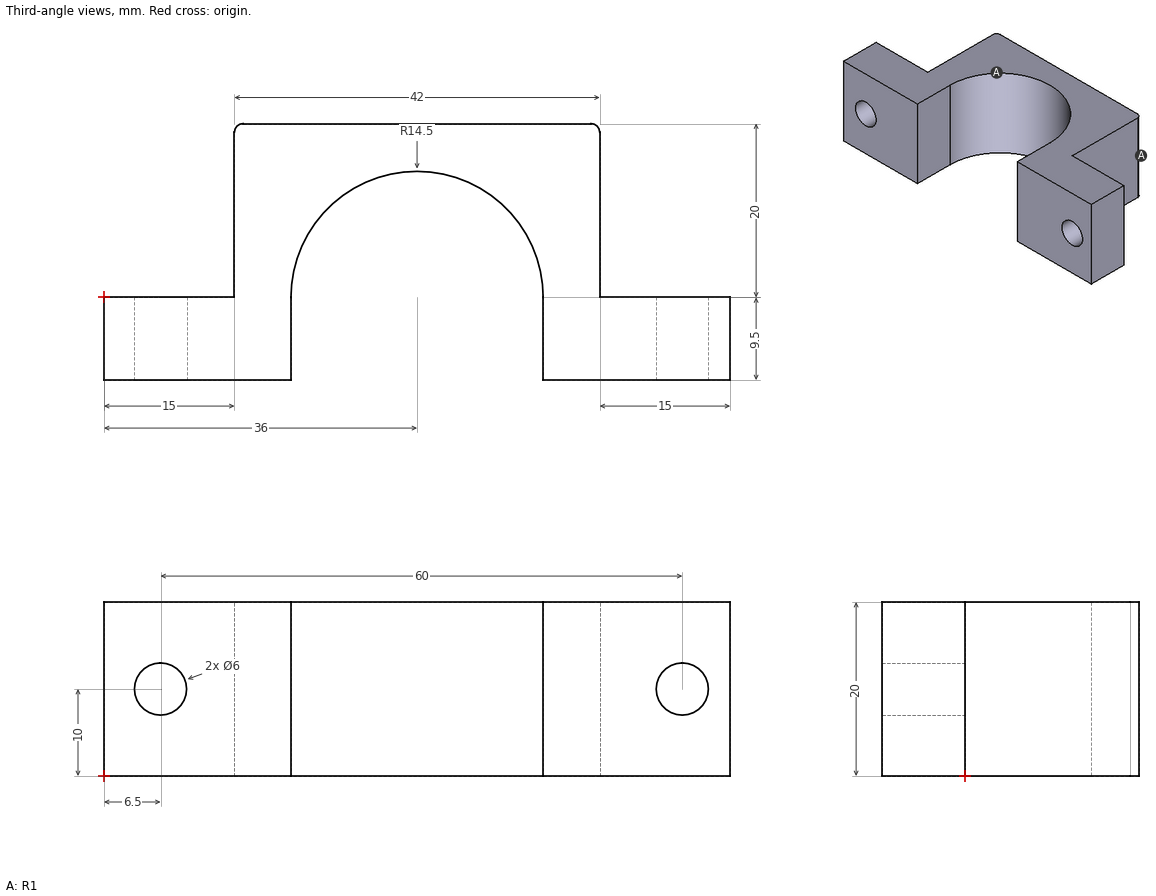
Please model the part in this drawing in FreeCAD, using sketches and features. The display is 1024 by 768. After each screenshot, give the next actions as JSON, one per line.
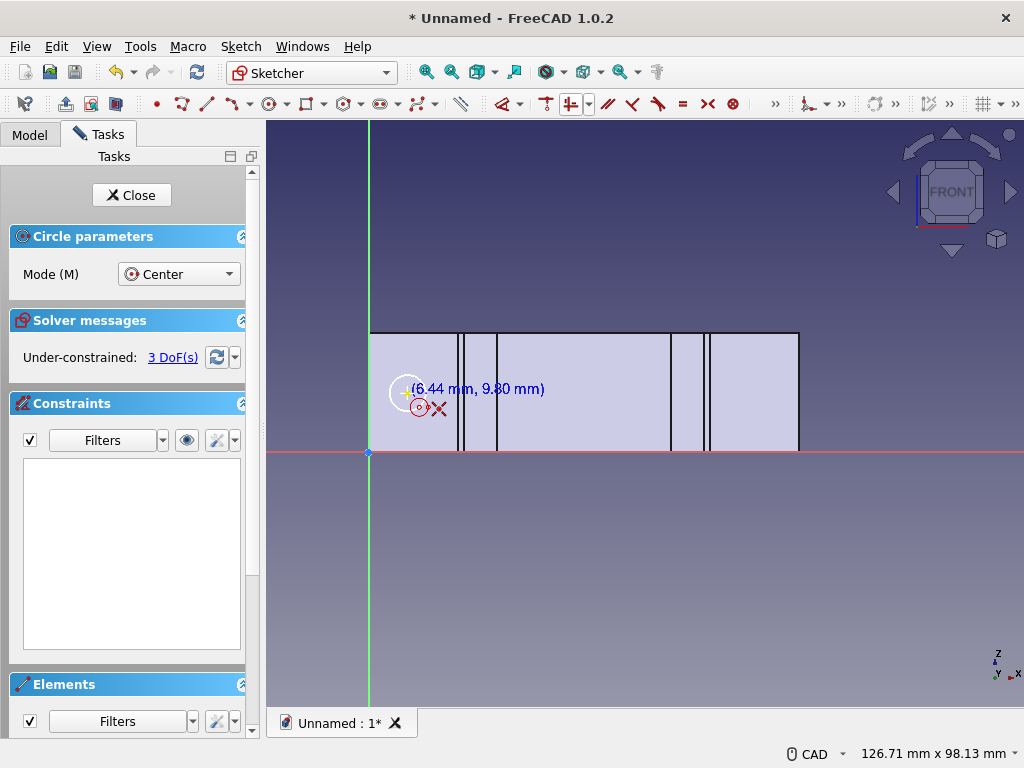
{"action": "scroll", "coordinate": [766, 393], "scroll_direction": "up", "scroll_amount": 2}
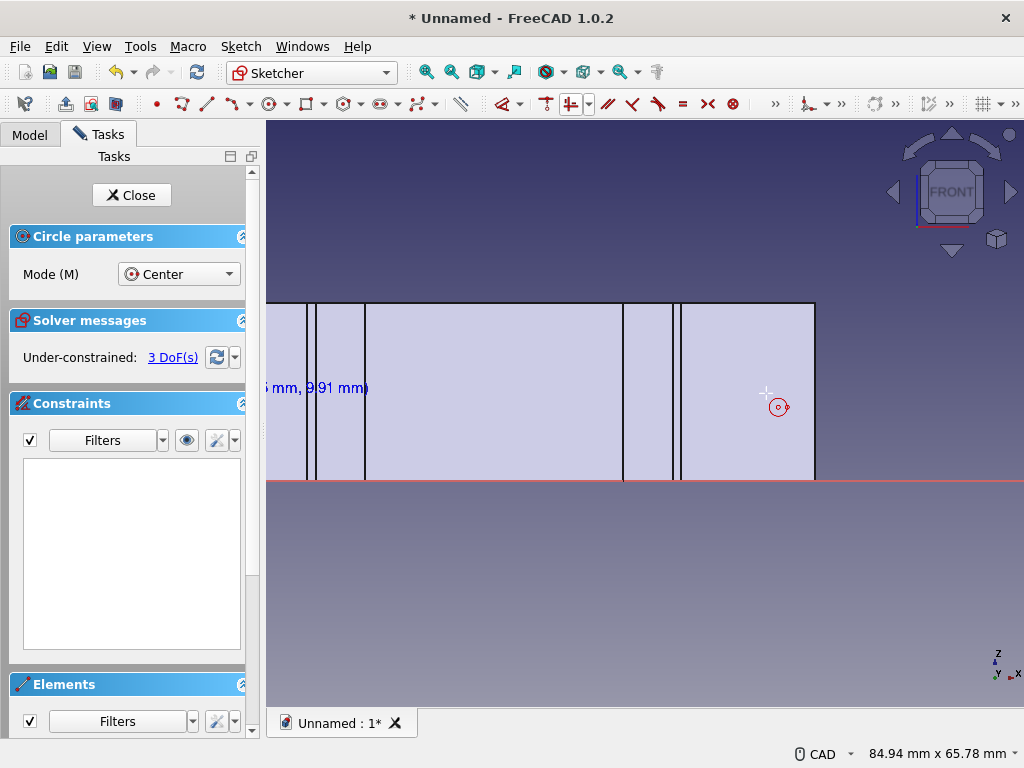
{"action": "left_click", "coordinate": [766, 392]}
{"action": "left_click", "coordinate": [785, 373]}
{"action": "key", "text": "Escape"}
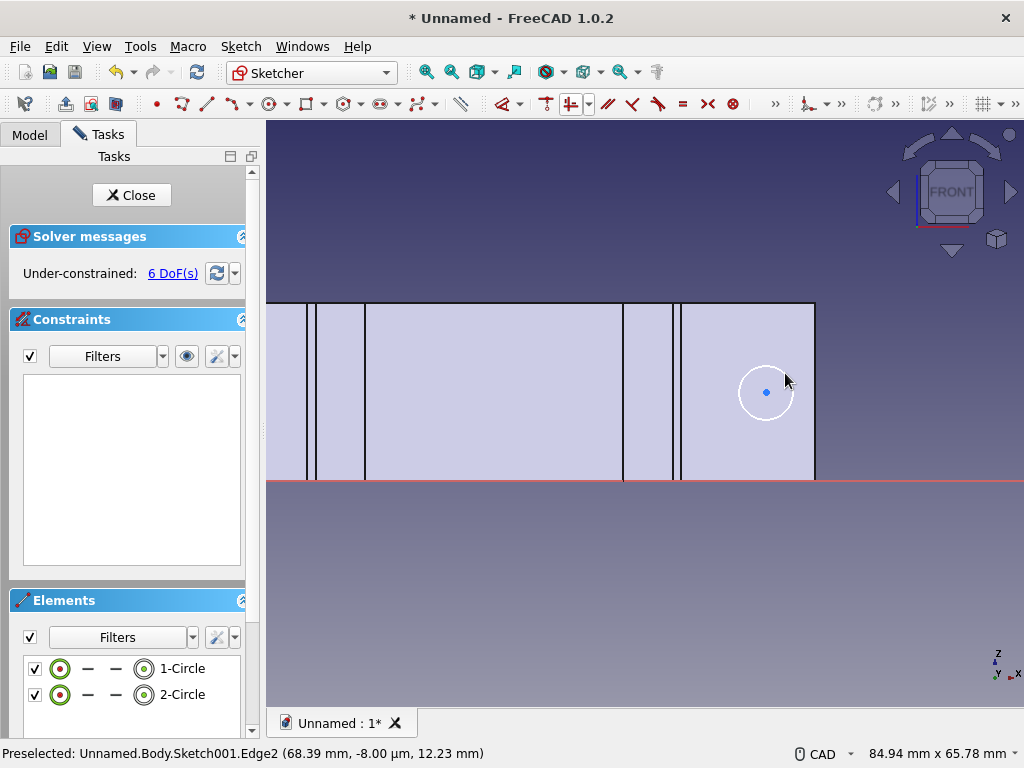
{"action": "scroll", "coordinate": [767, 393], "scroll_direction": "down", "scroll_amount": 2}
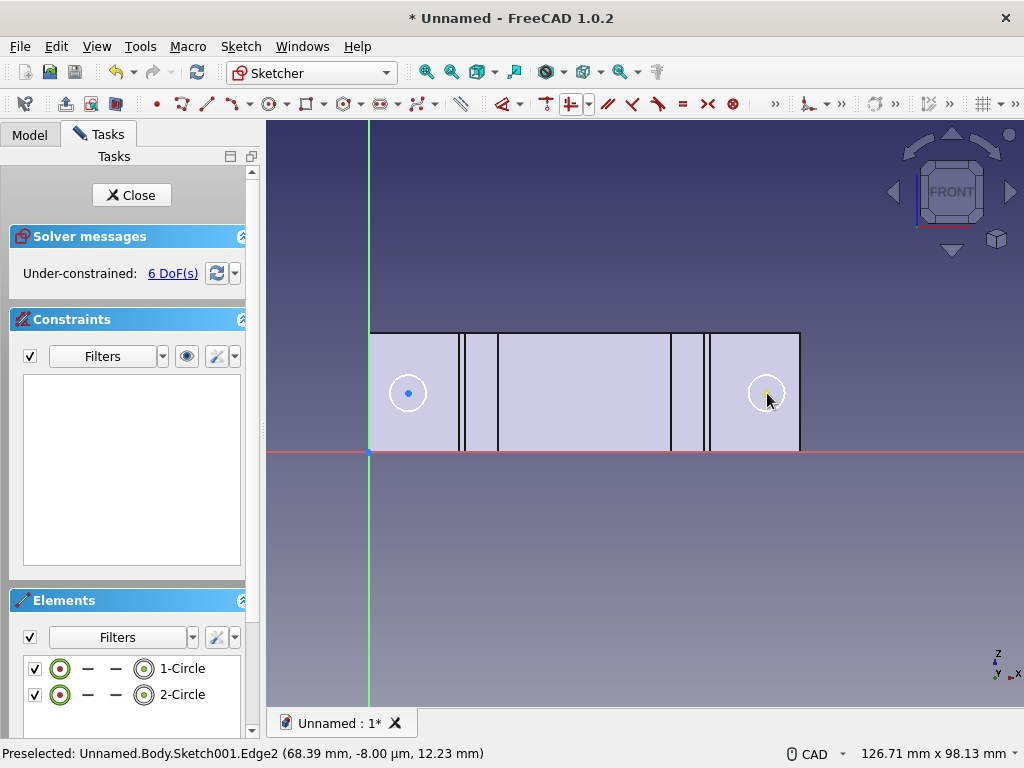
{"action": "left_click", "coordinate": [421, 380]}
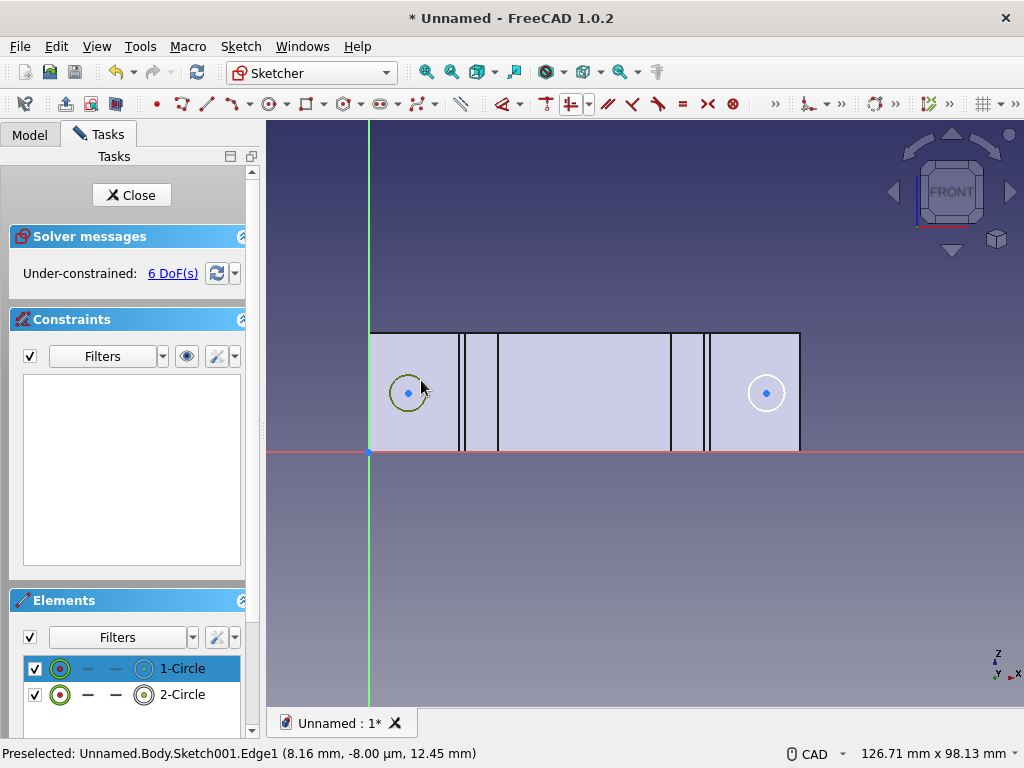
{"action": "left_click", "coordinate": [779, 380]}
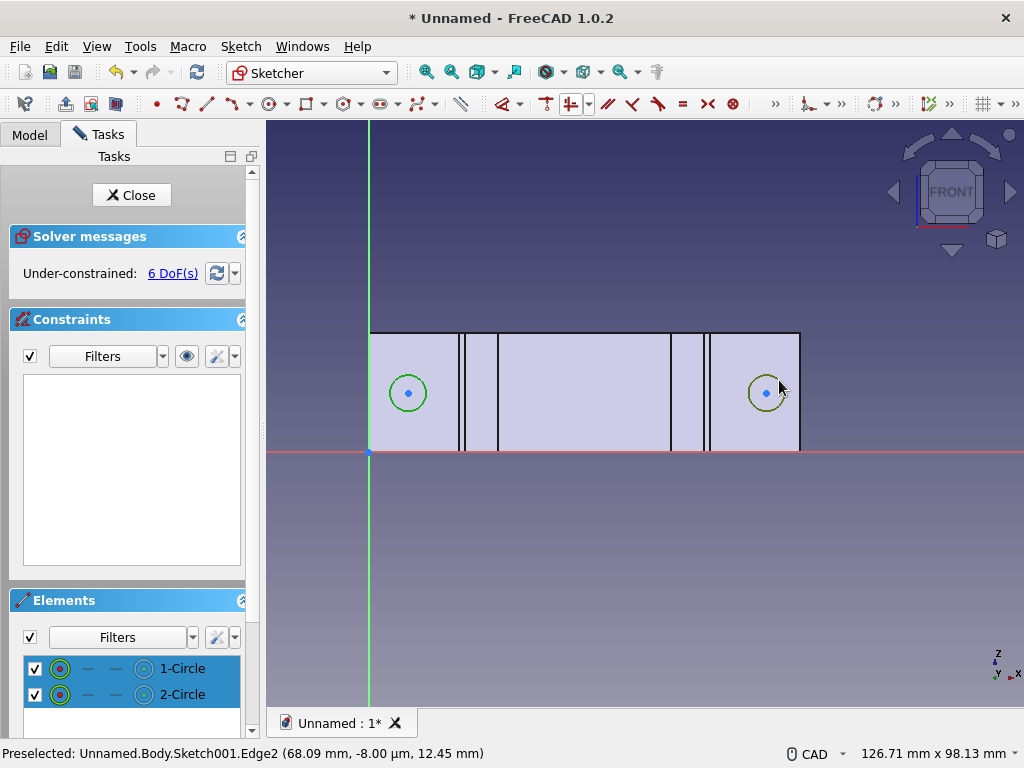
{"action": "left_click", "coordinate": [683, 104]}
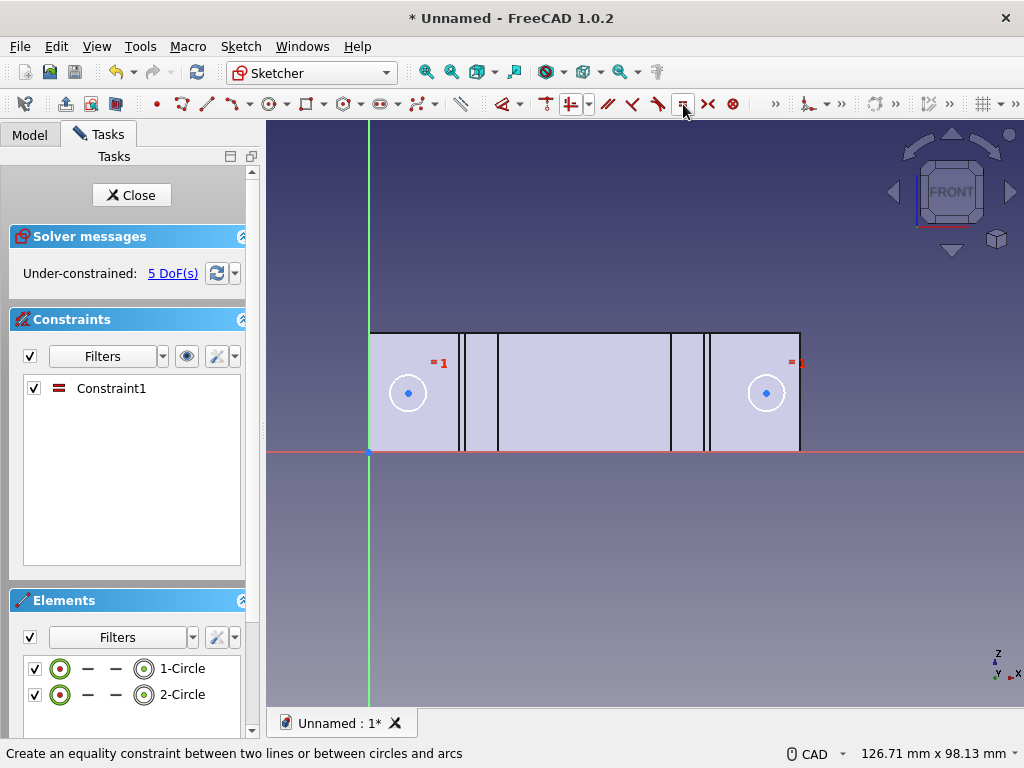
{"action": "left_click", "coordinate": [502, 104]}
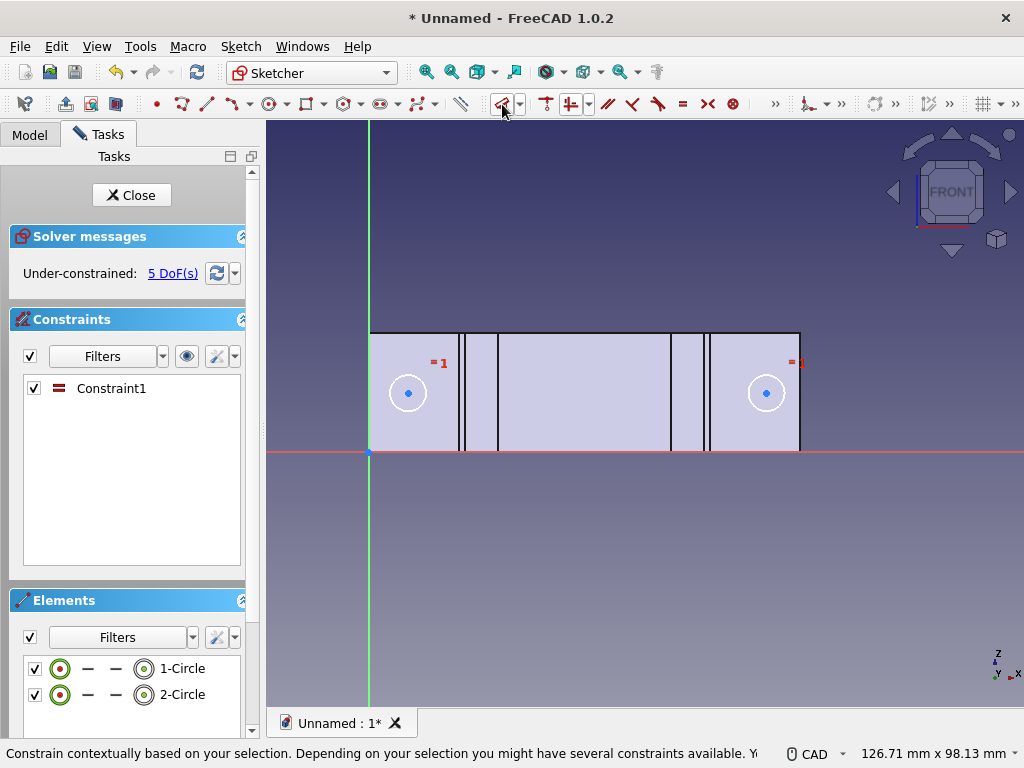
{"action": "left_click", "coordinate": [421, 380]}
{"action": "left_click", "coordinate": [443, 357]}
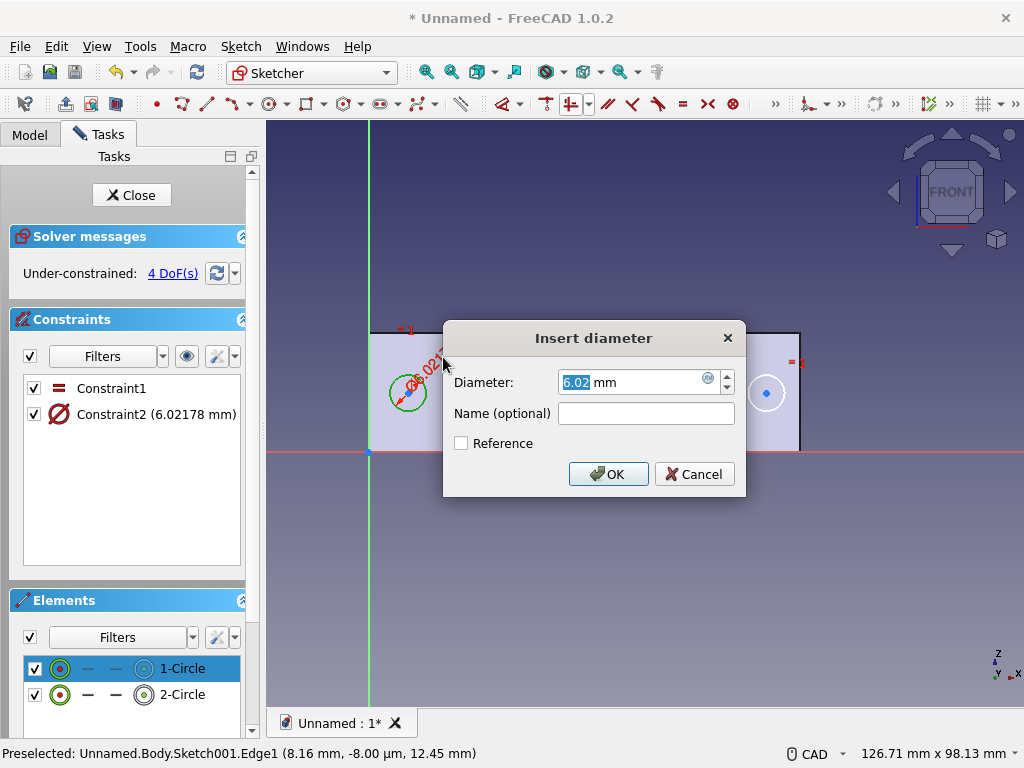
{"action": "type", "text": "6"}
{"action": "key", "text": "Return"}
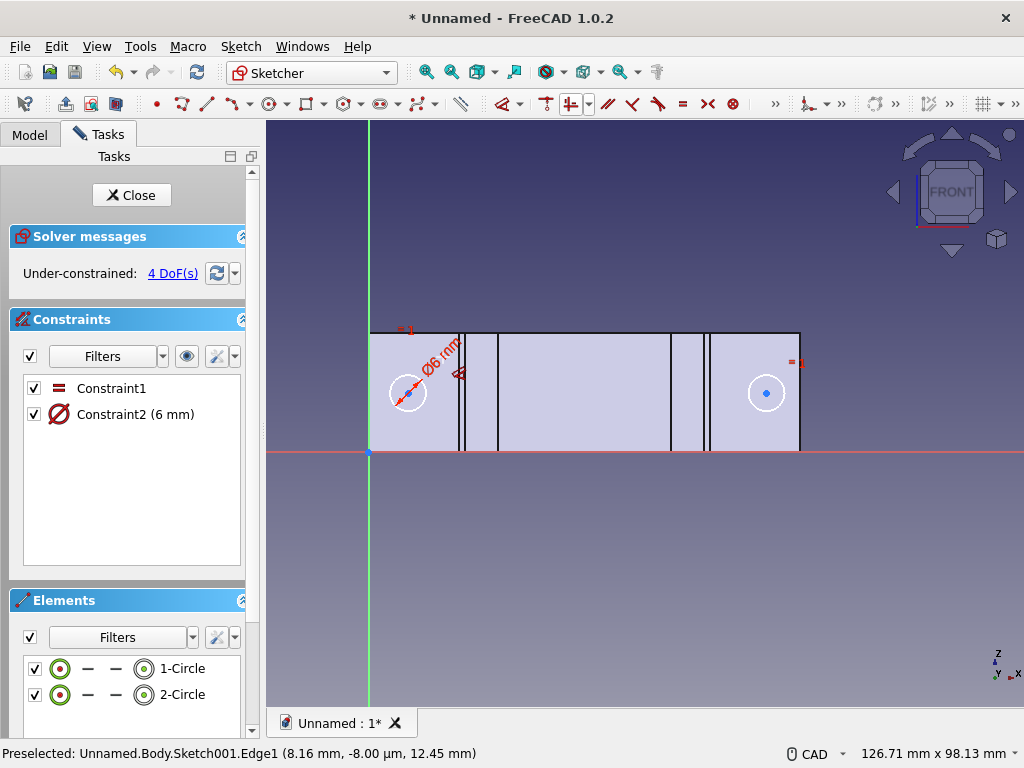
{"action": "left_click", "coordinate": [408, 393]}
{"action": "left_click", "coordinate": [335, 423]}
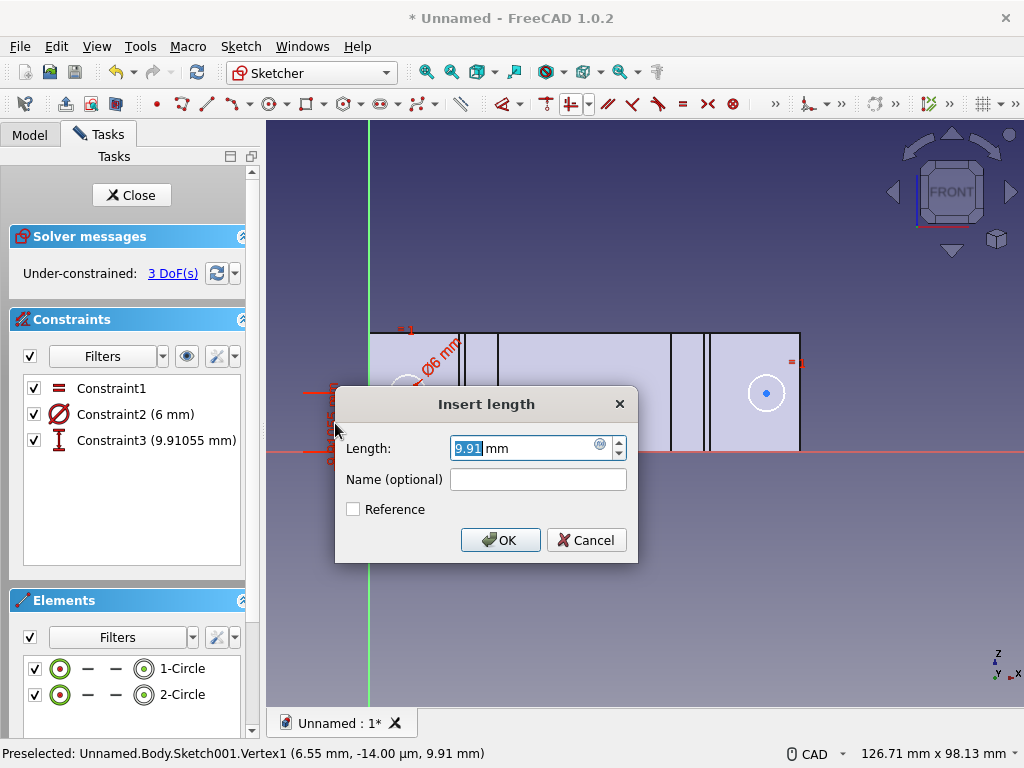
{"action": "type", "text": "10"}
{"action": "key", "text": "Return"}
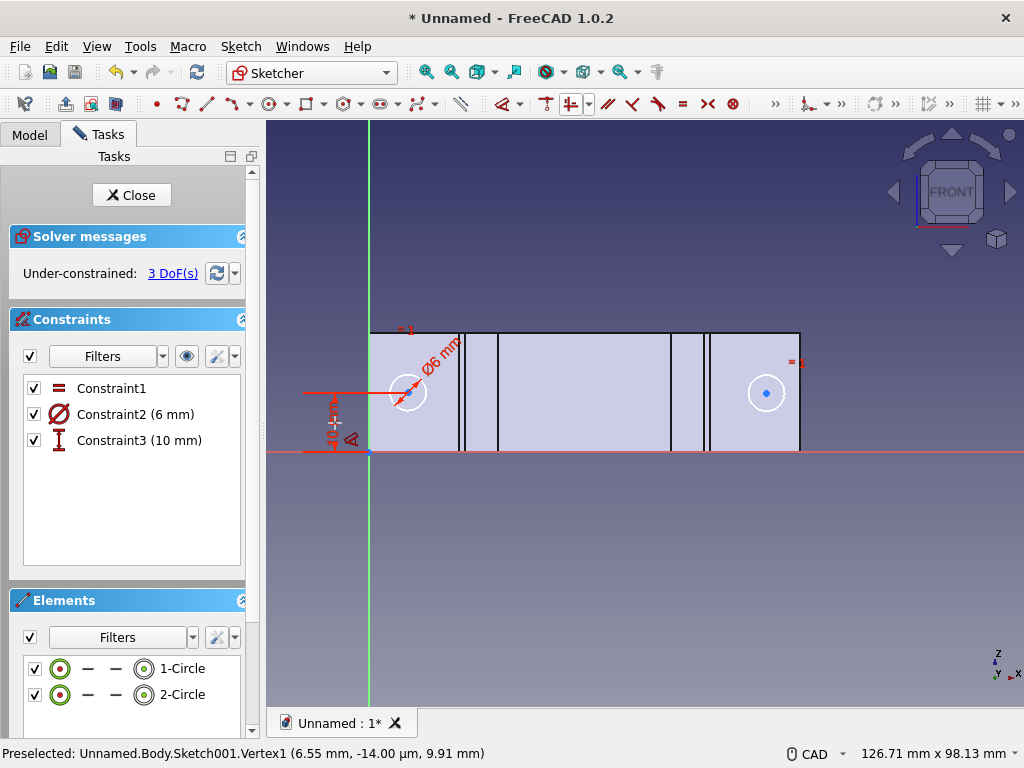
{"action": "left_click", "coordinate": [767, 393]}
{"action": "left_click", "coordinate": [335, 402]}